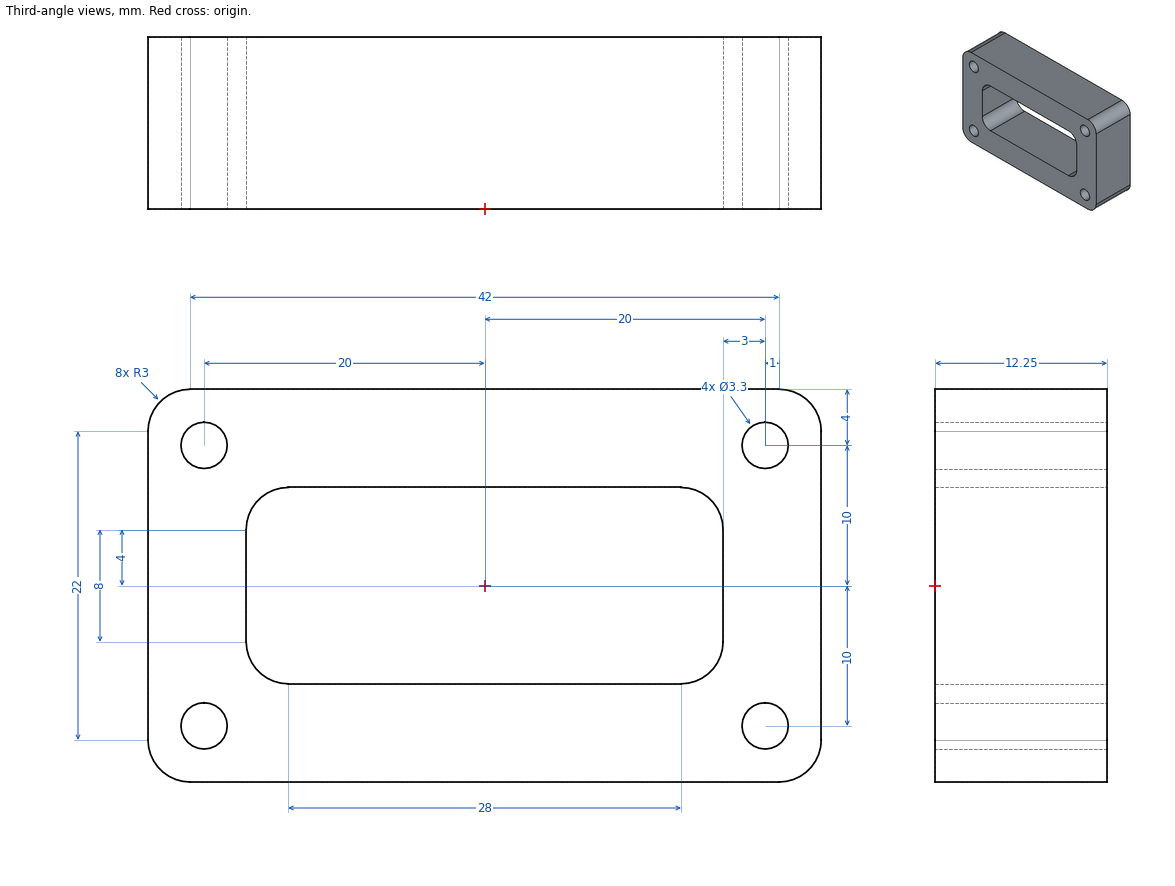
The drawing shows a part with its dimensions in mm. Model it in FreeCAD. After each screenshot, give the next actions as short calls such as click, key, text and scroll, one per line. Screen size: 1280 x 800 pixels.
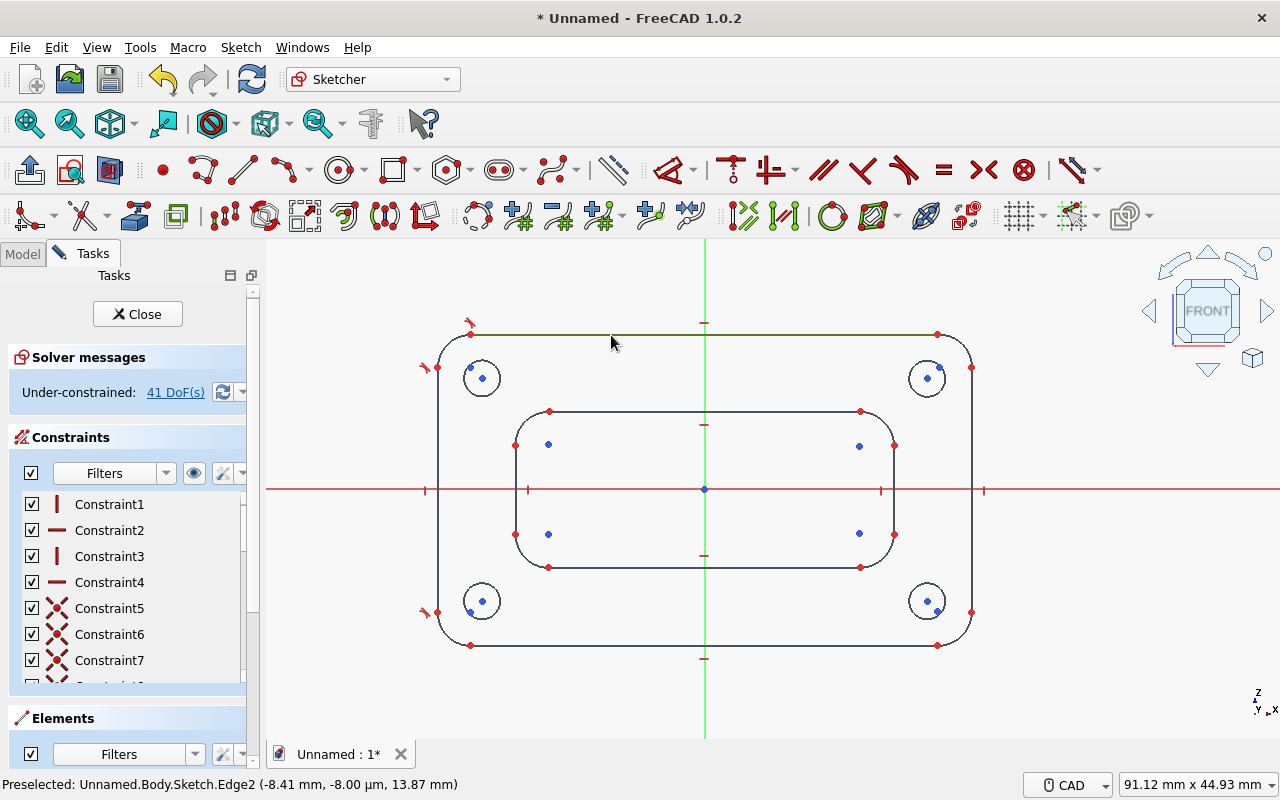
click(968, 352)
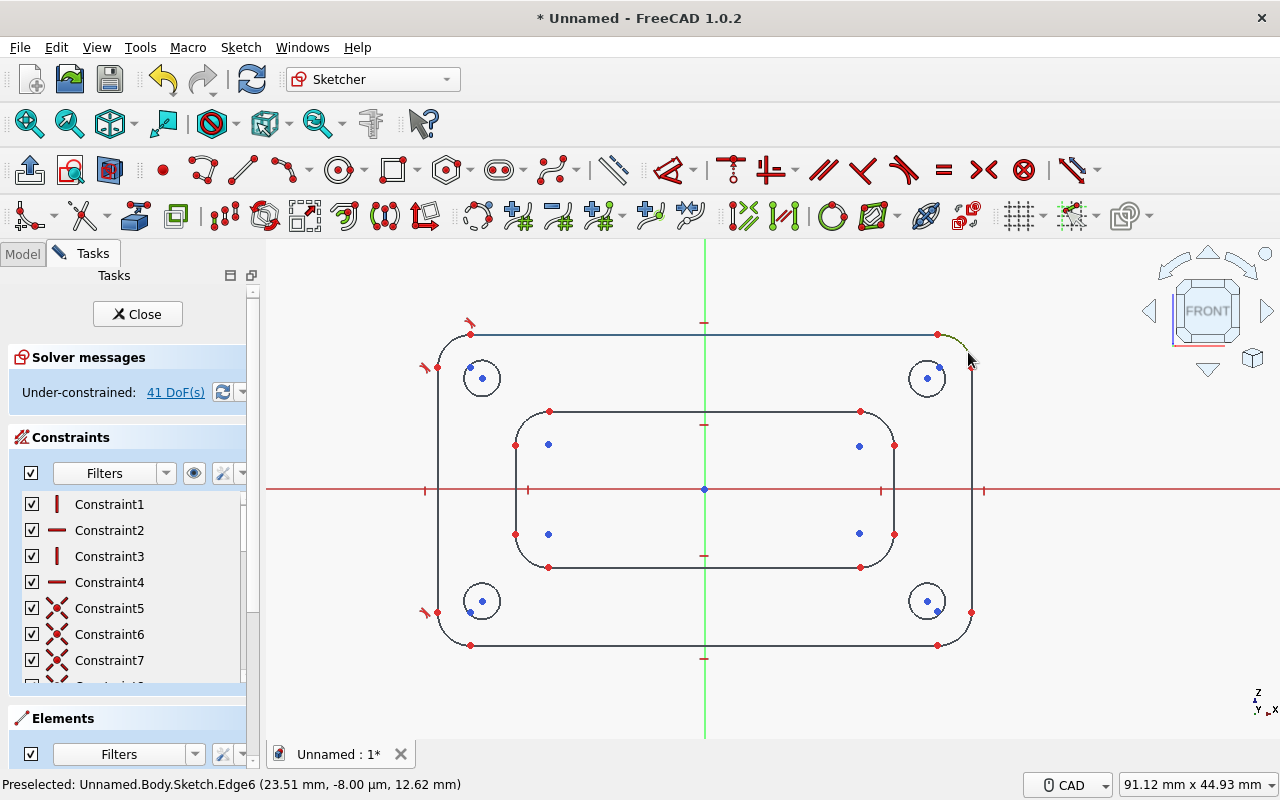
click(904, 170)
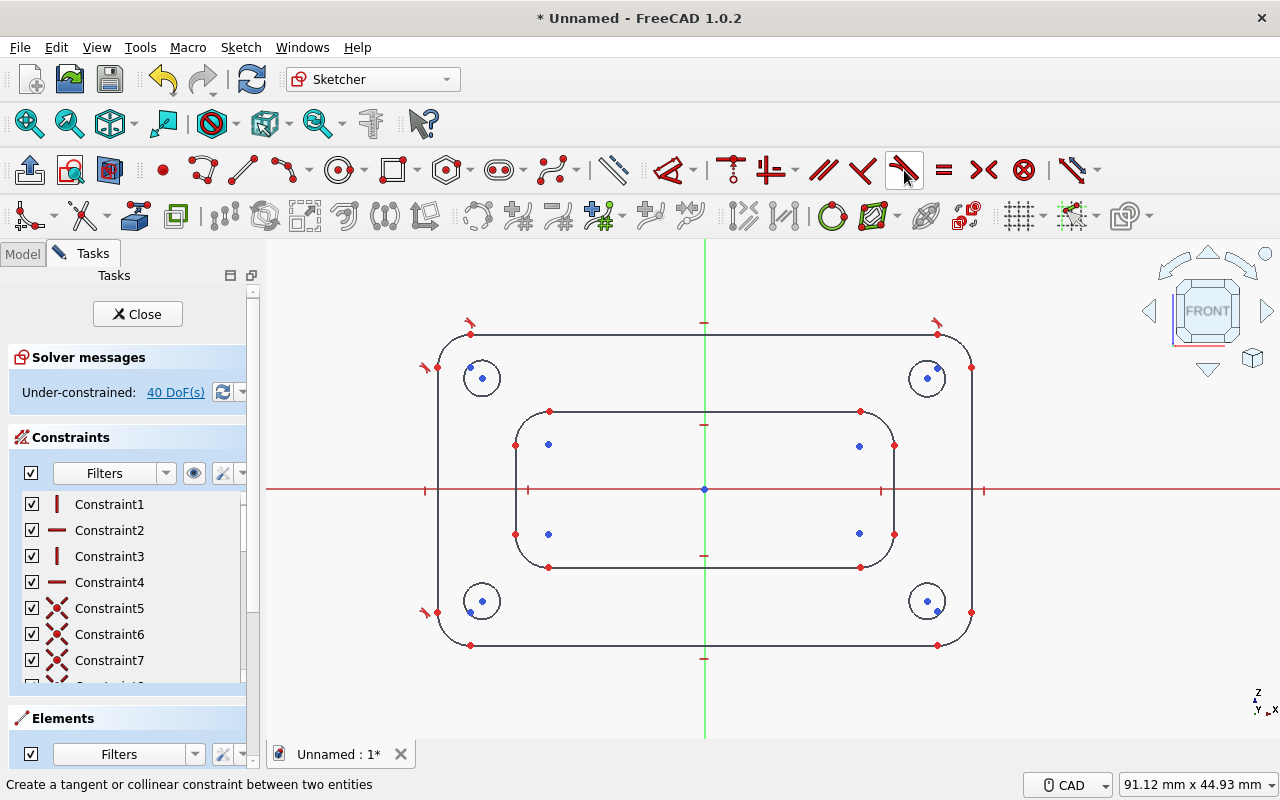
click(972, 441)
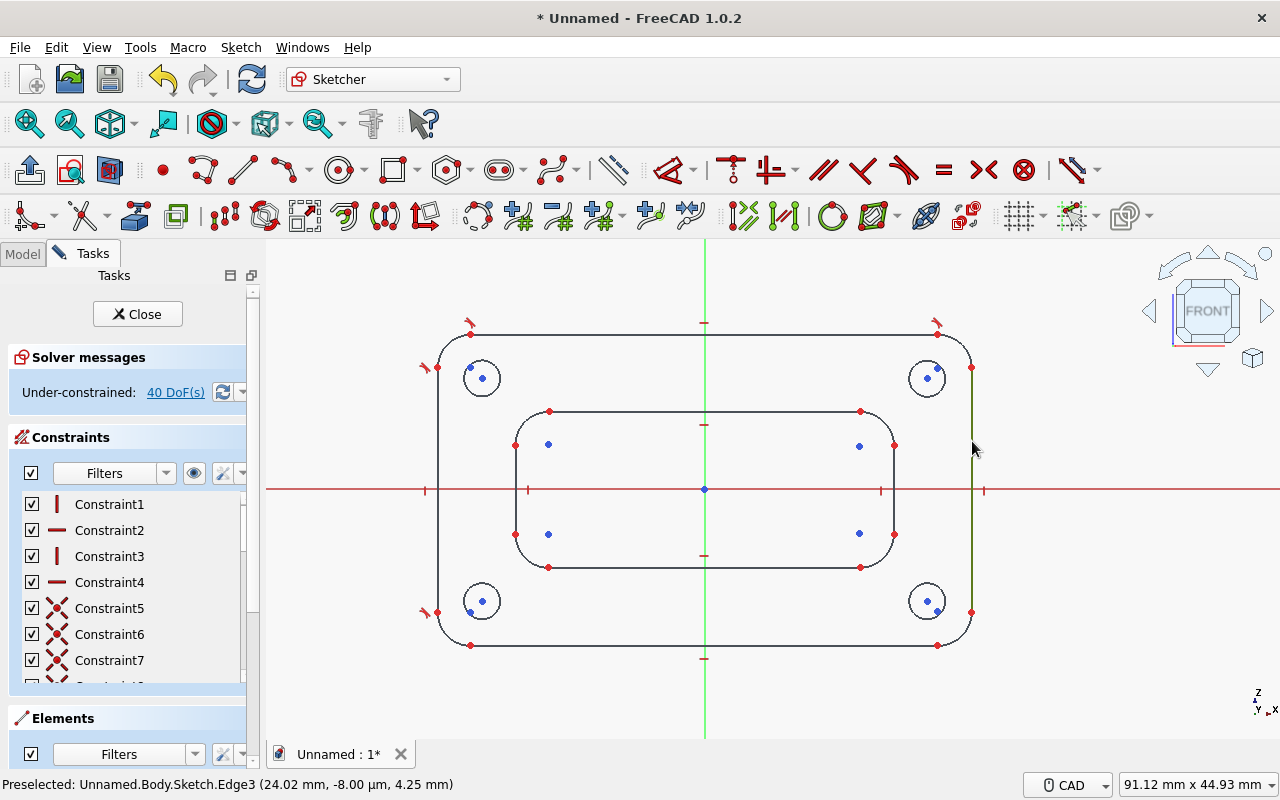
click(968, 353)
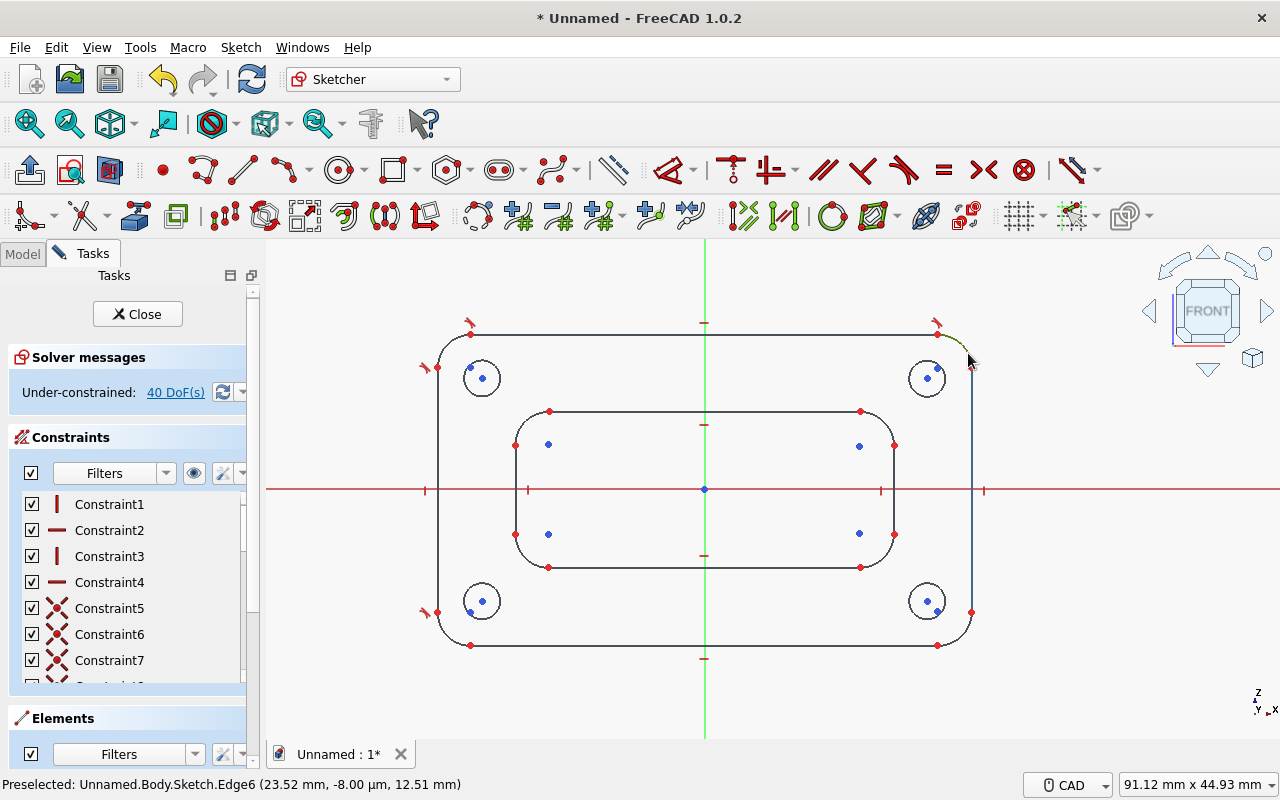
click(904, 170)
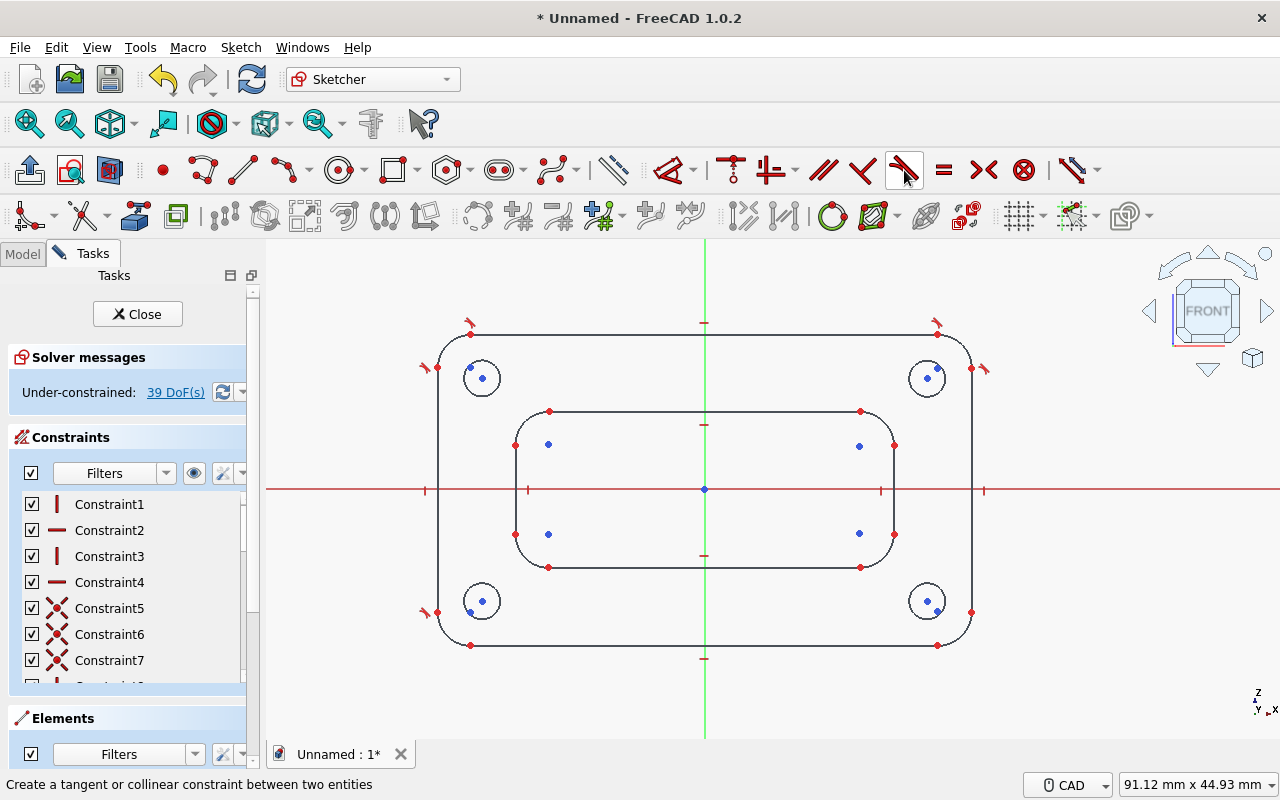
click(972, 442)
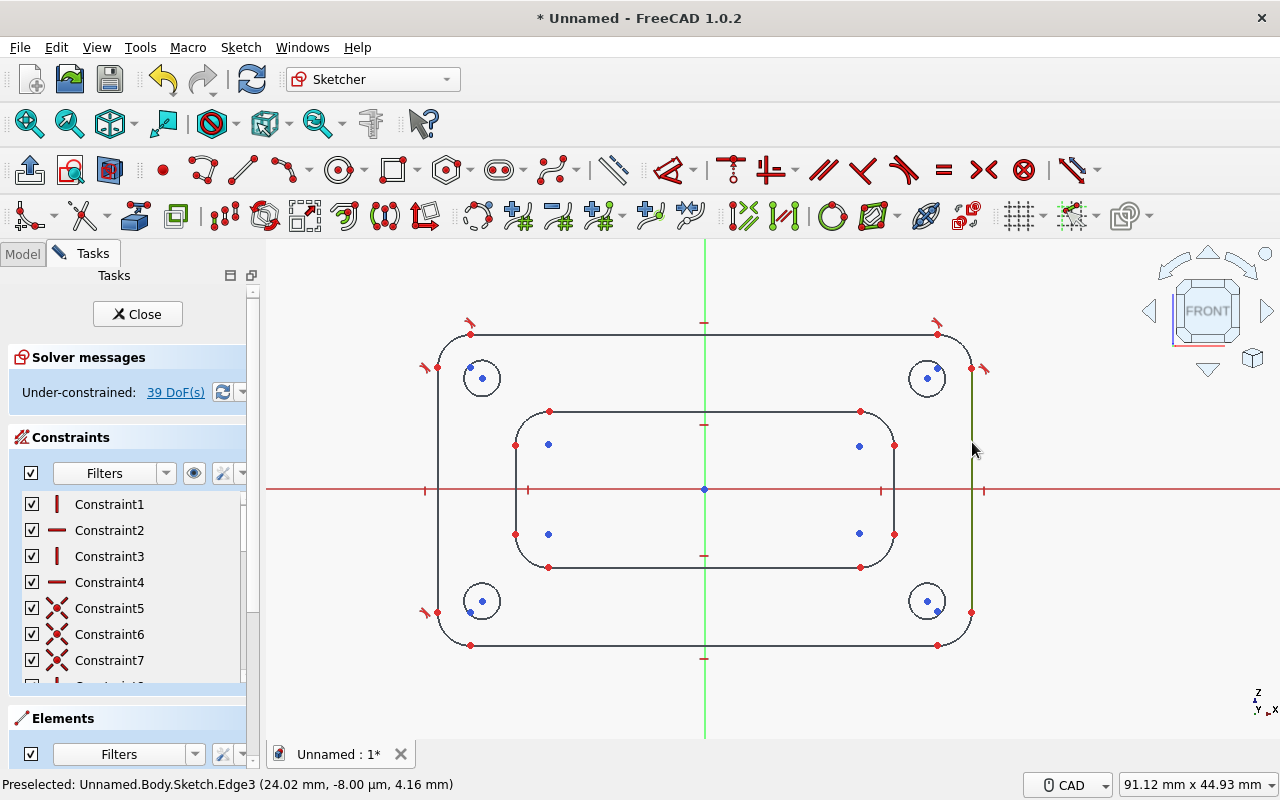
click(953, 642)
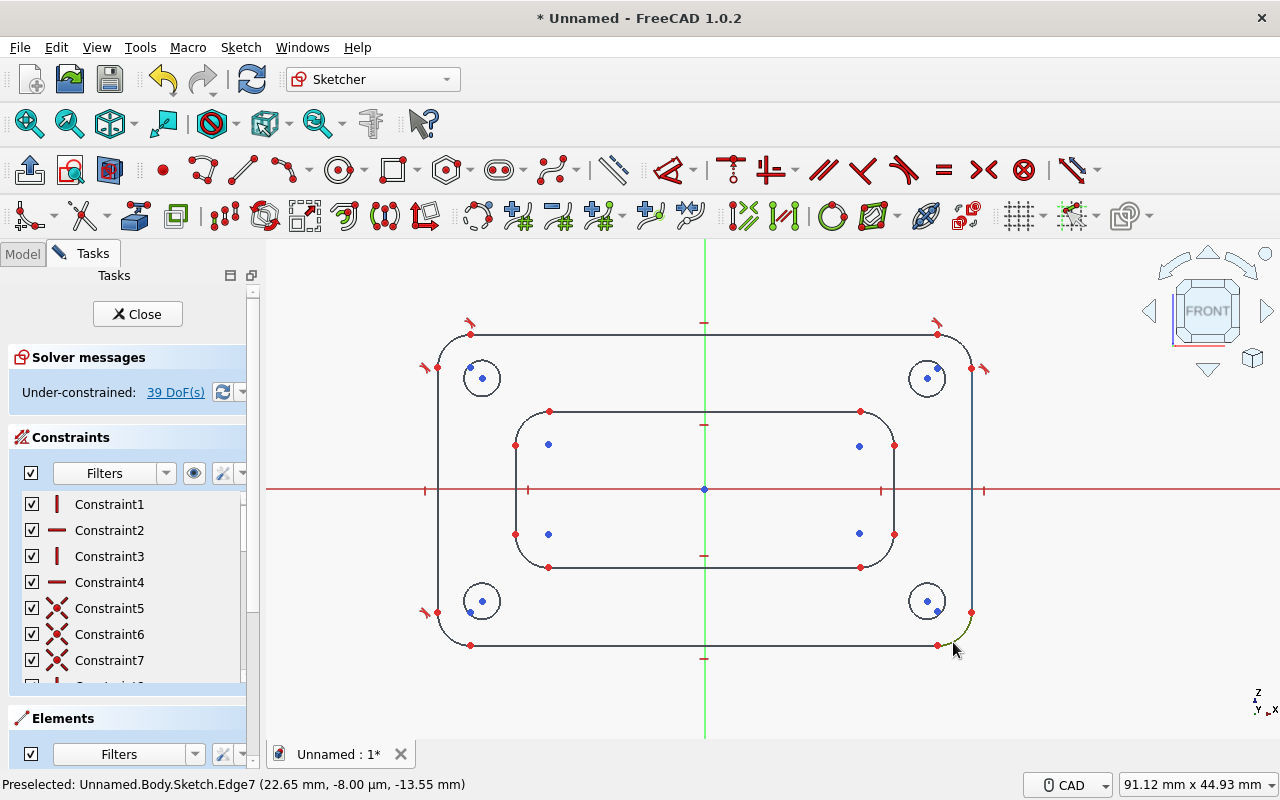
click(904, 170)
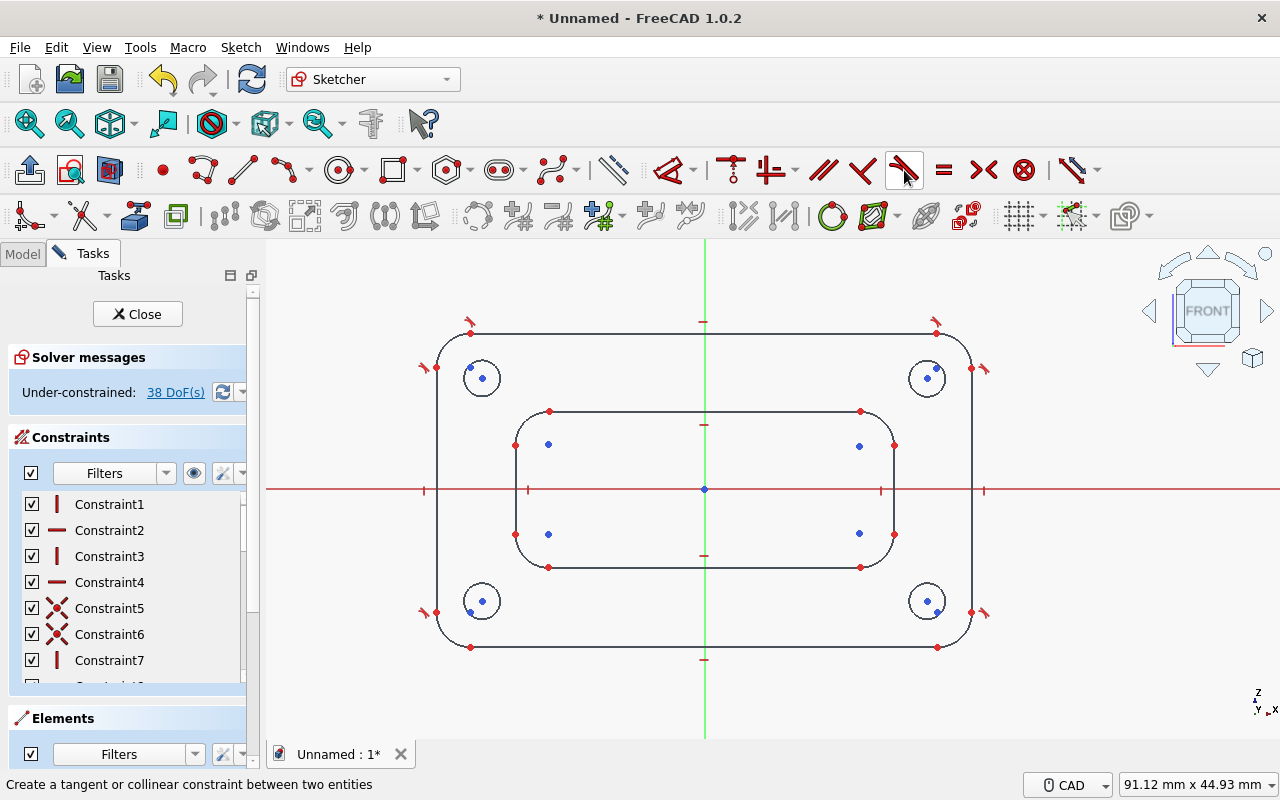
click(798, 647)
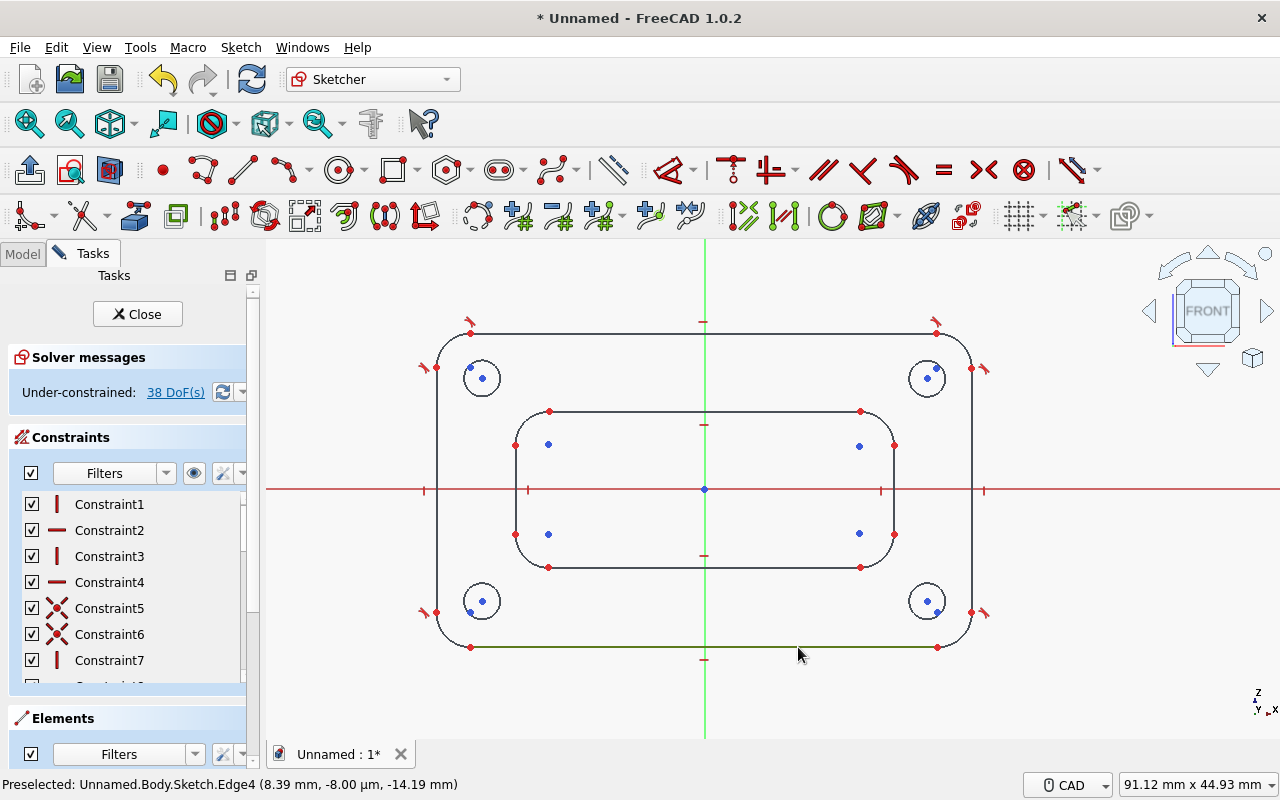
click(953, 643)